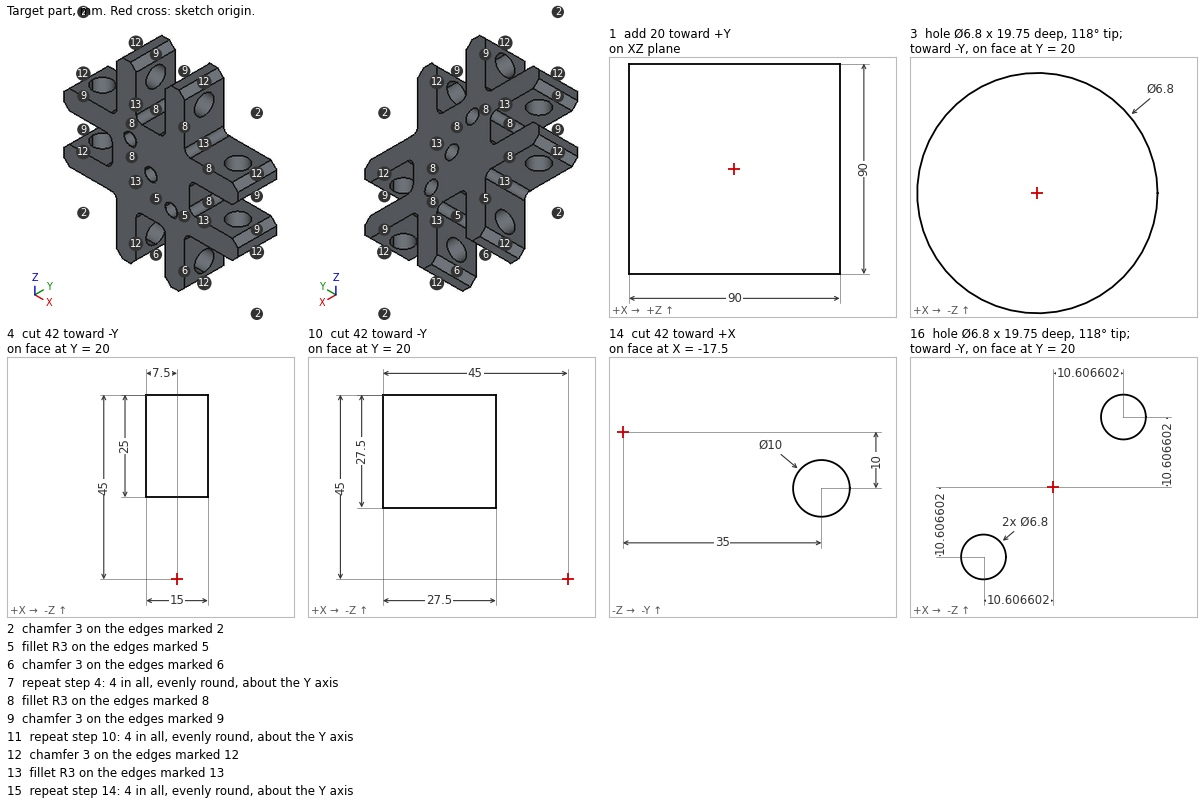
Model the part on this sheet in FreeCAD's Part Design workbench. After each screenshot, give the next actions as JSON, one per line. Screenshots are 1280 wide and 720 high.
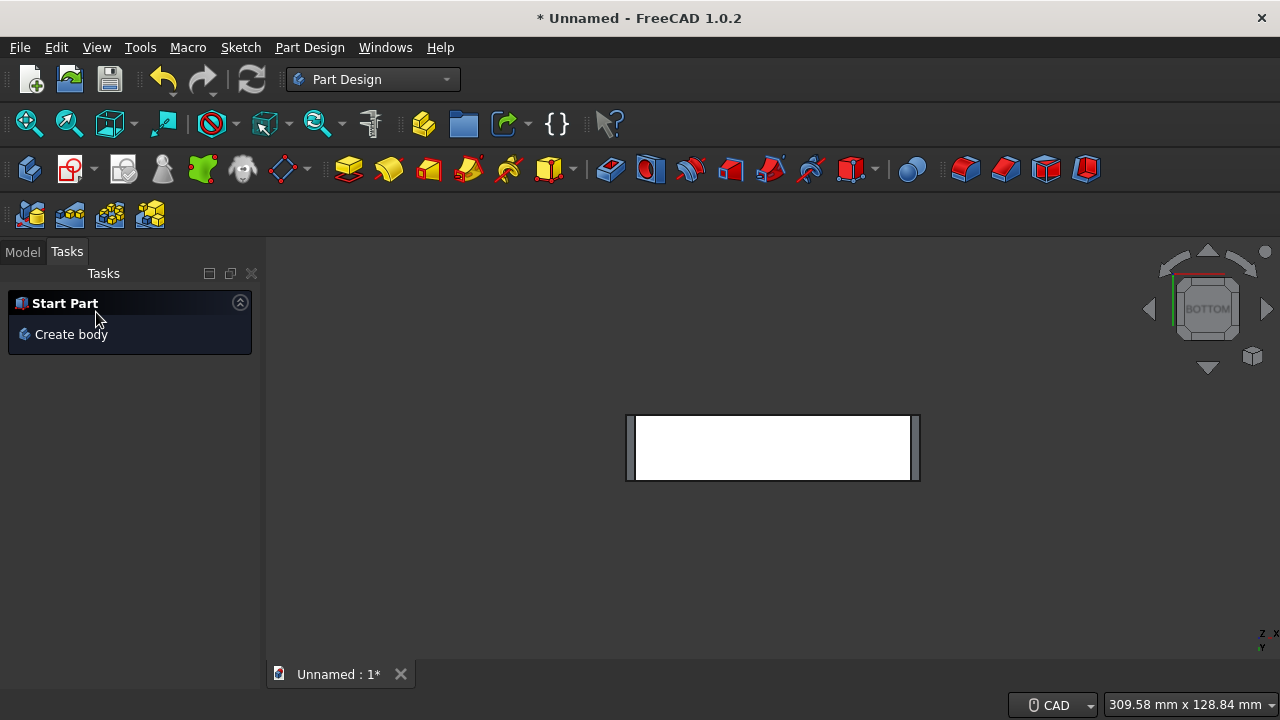
{"action": "left_click", "coordinate": [30, 124]}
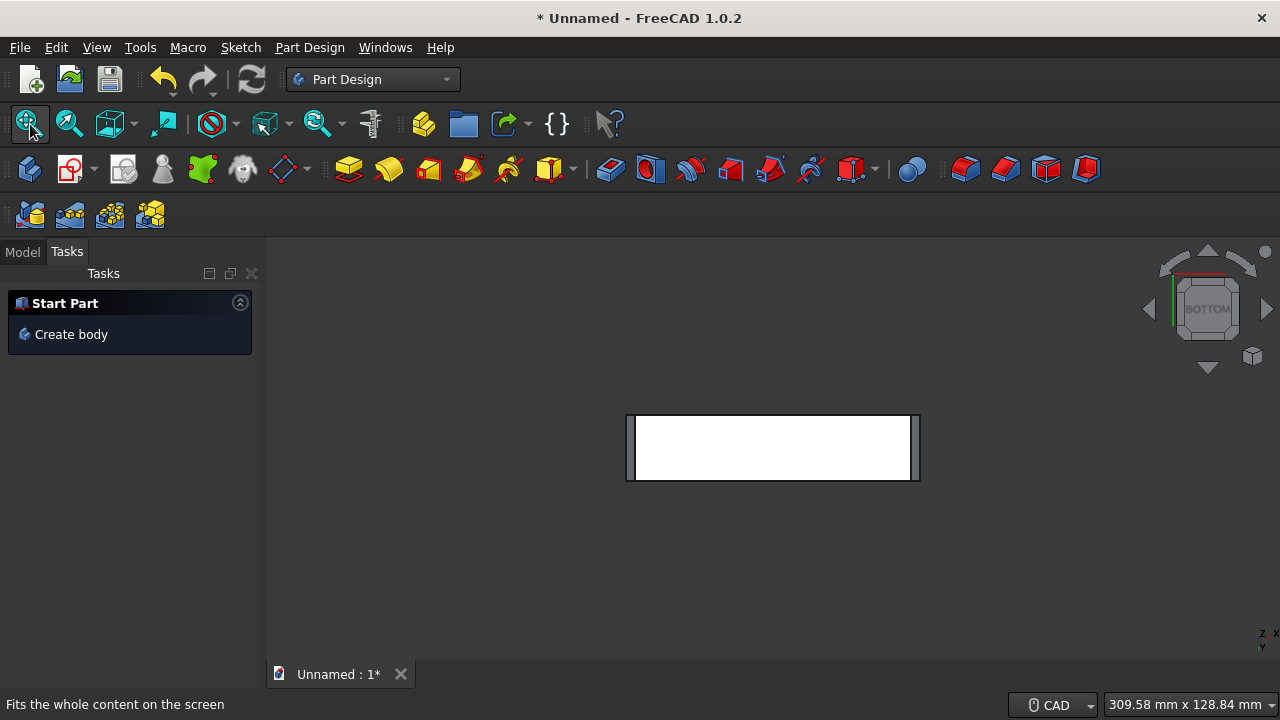
{"action": "key", "text": "4"}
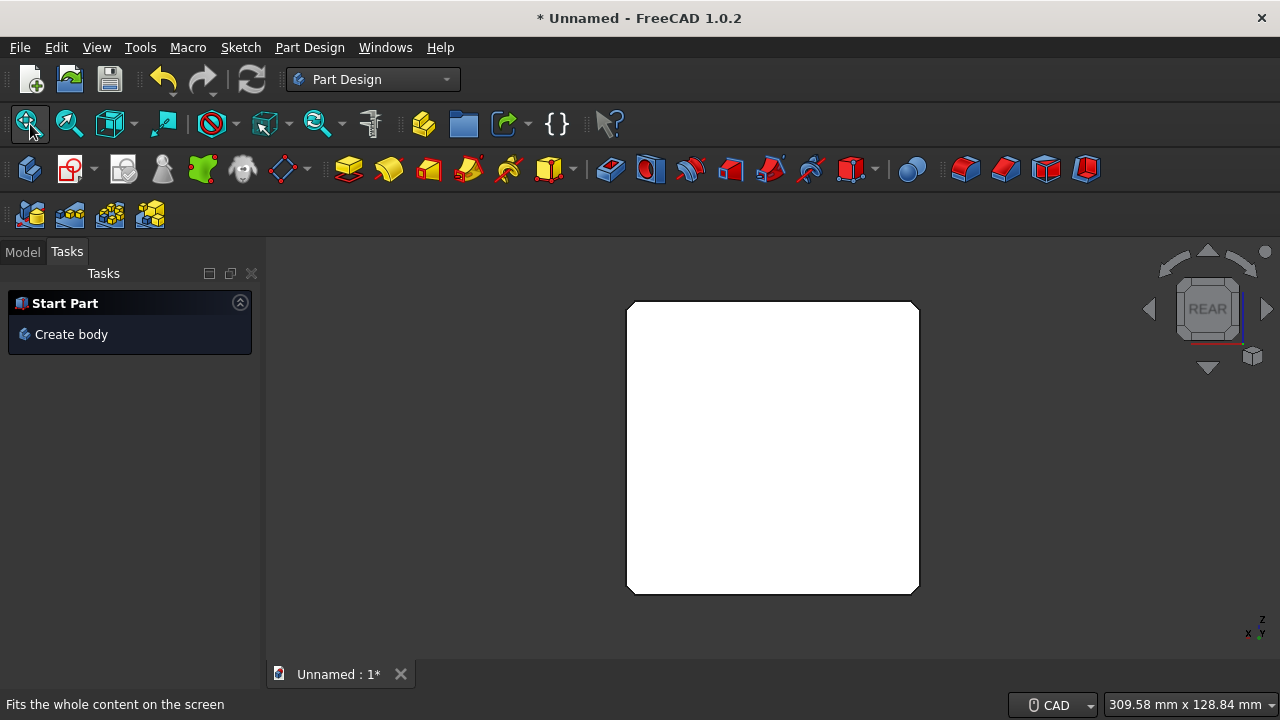
{"action": "left_click", "coordinate": [773, 447]}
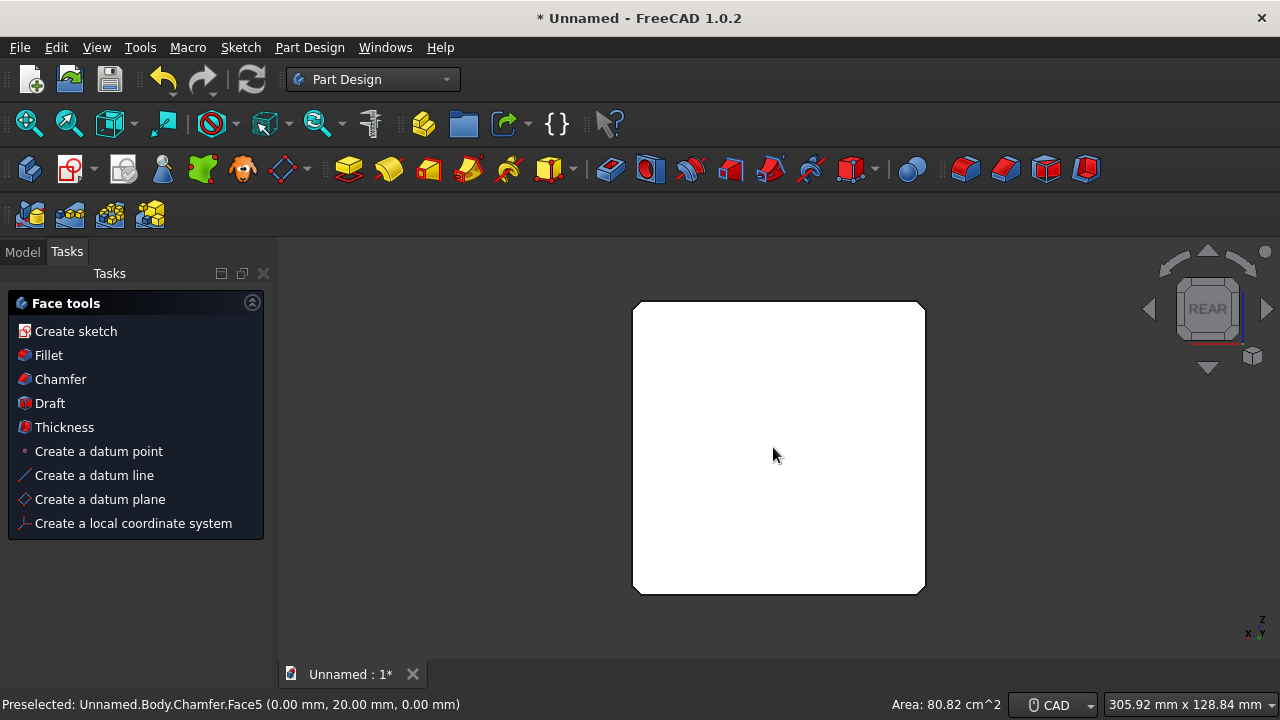
{"action": "left_click", "coordinate": [70, 170]}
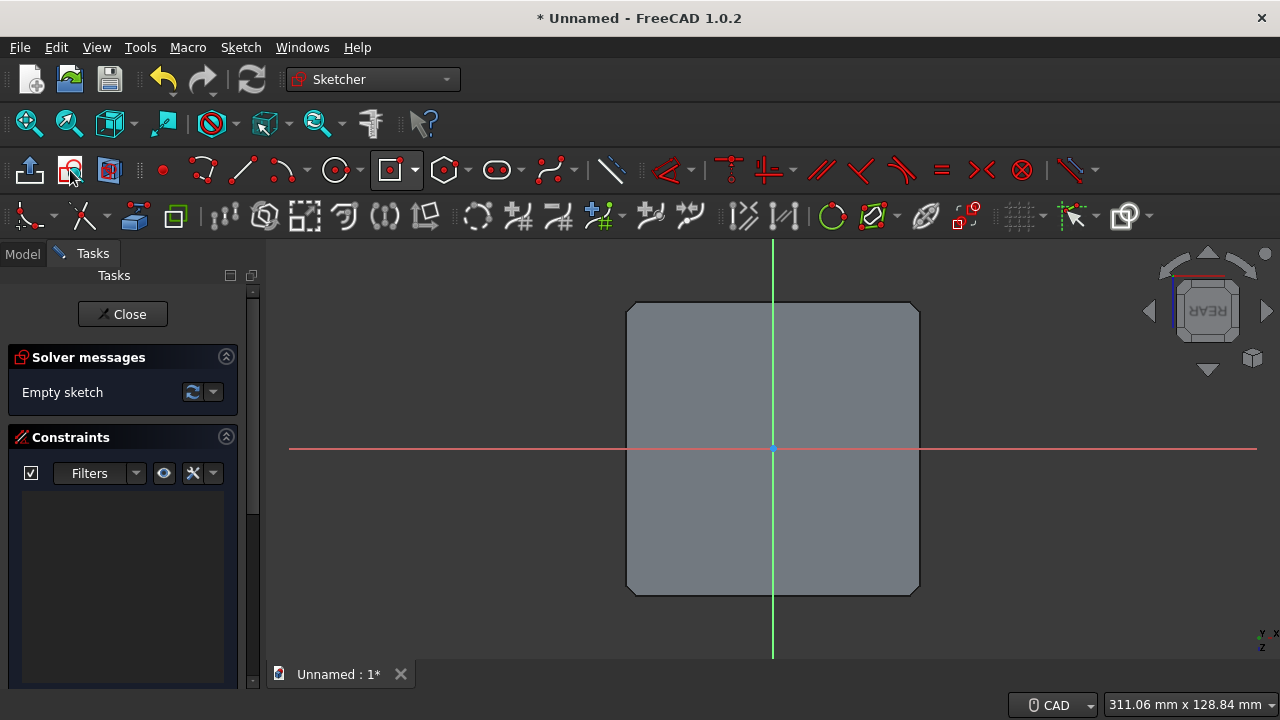
{"action": "scroll", "coordinate": [780, 449], "scroll_direction": "up", "scroll_amount": 12}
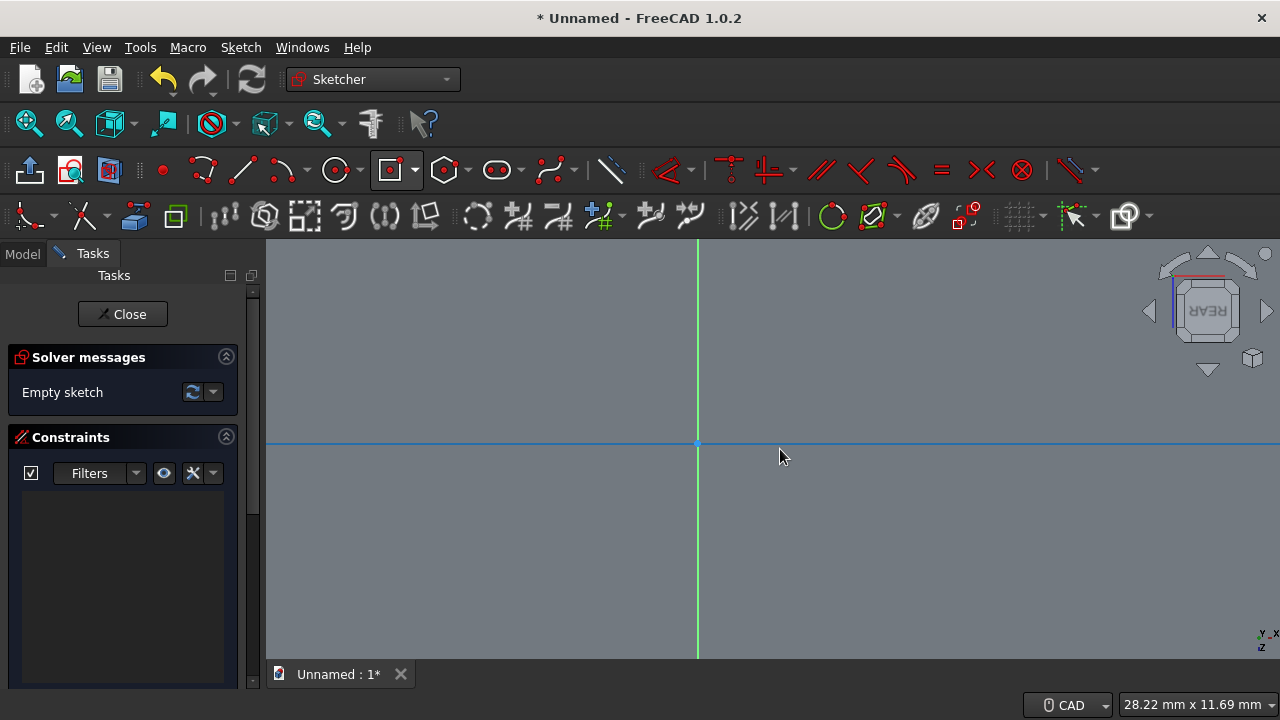
{"action": "left_click", "coordinate": [336, 170]}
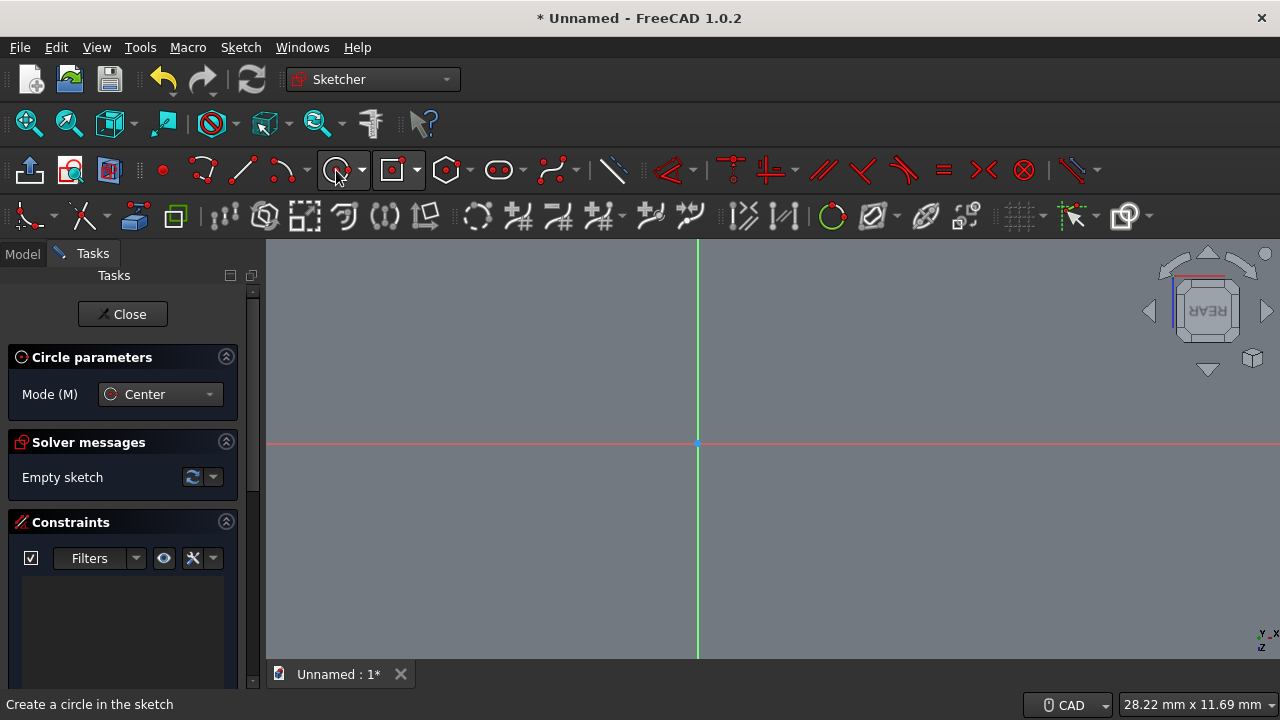
{"action": "left_click", "coordinate": [698, 444]}
{"action": "left_click", "coordinate": [784, 358]}
{"action": "key", "text": "Escape"}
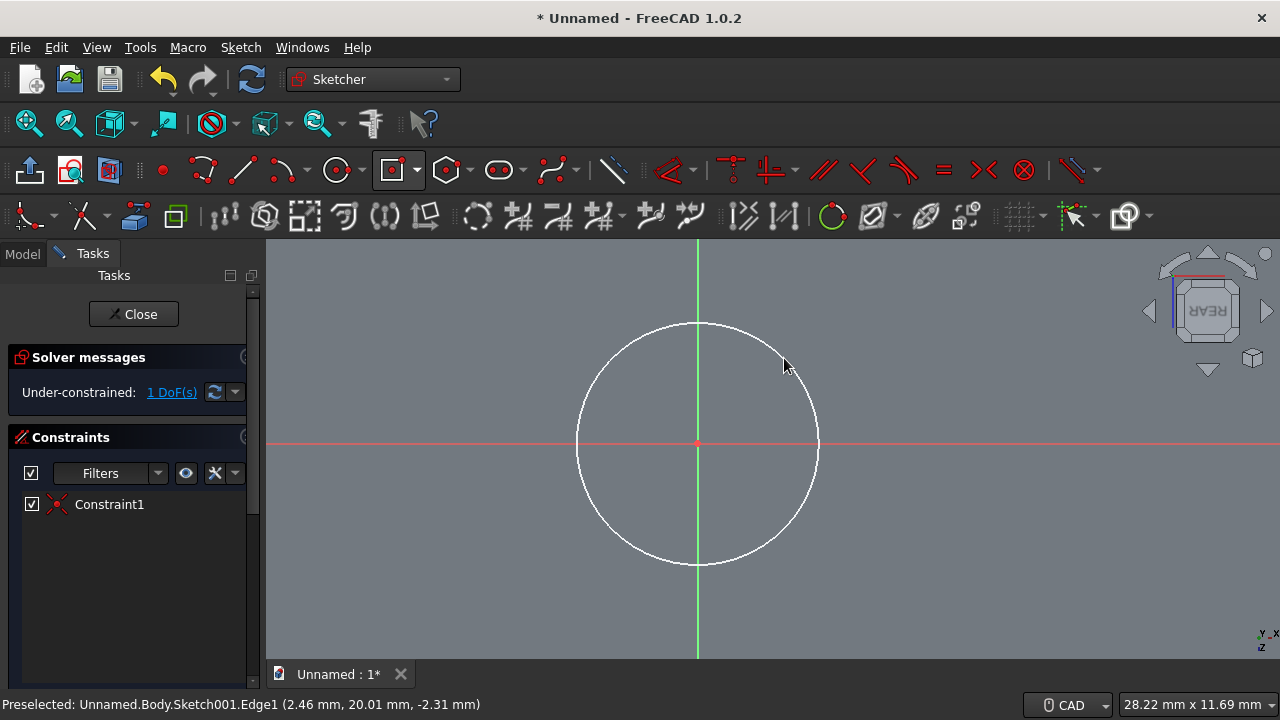
{"action": "left_click", "coordinate": [668, 170]}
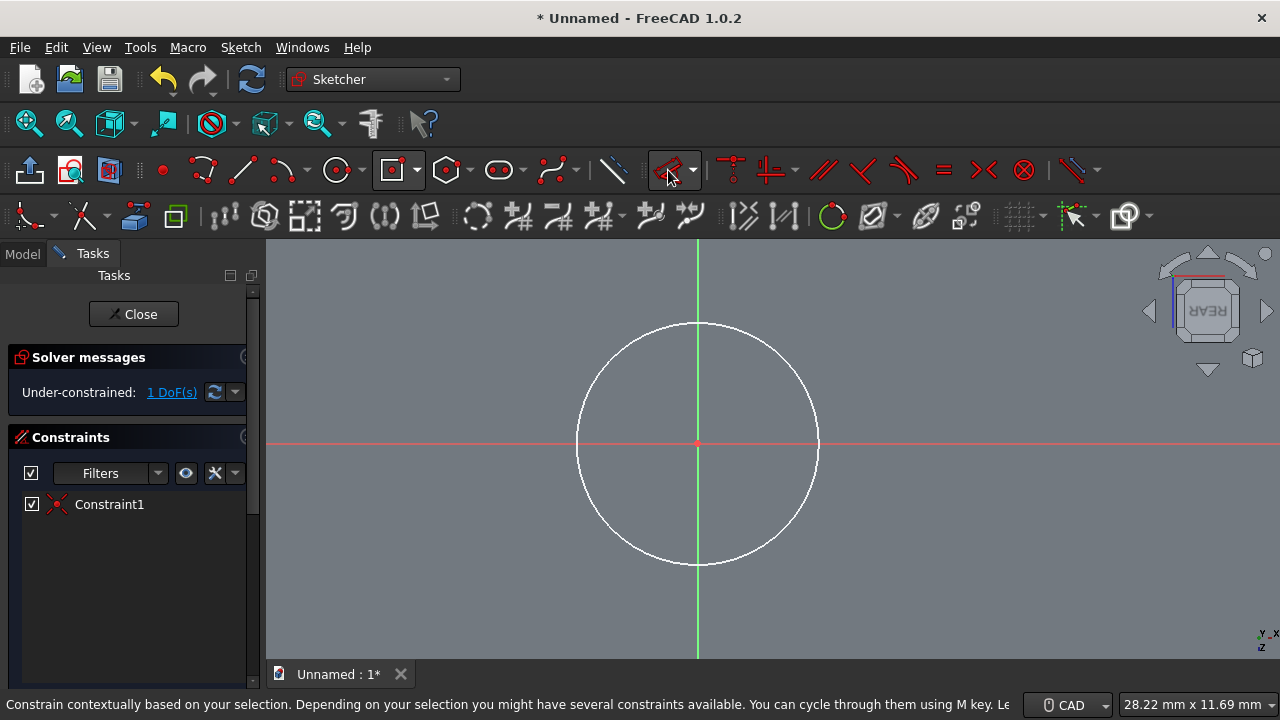
{"action": "left_click", "coordinate": [783, 358]}
{"action": "left_click", "coordinate": [806, 335]}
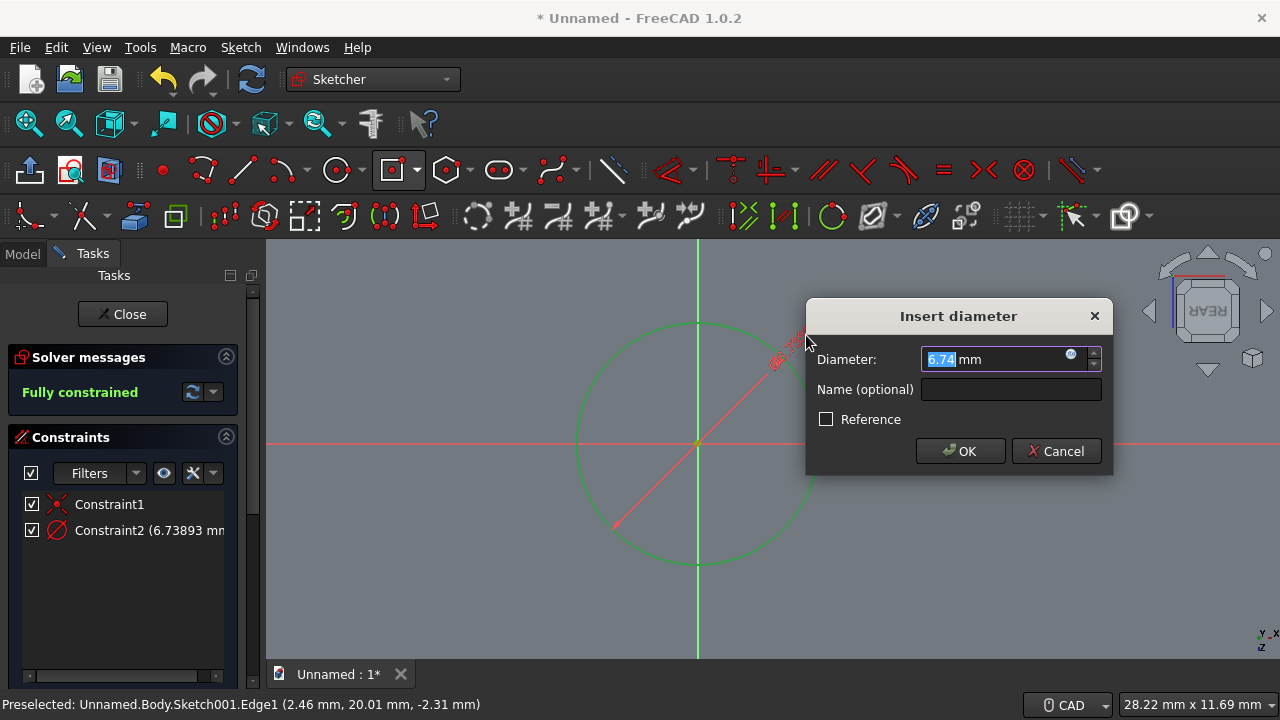
{"action": "type", "text": "6.8"}
{"action": "key", "text": "Return"}
{"action": "key", "text": "Escape"}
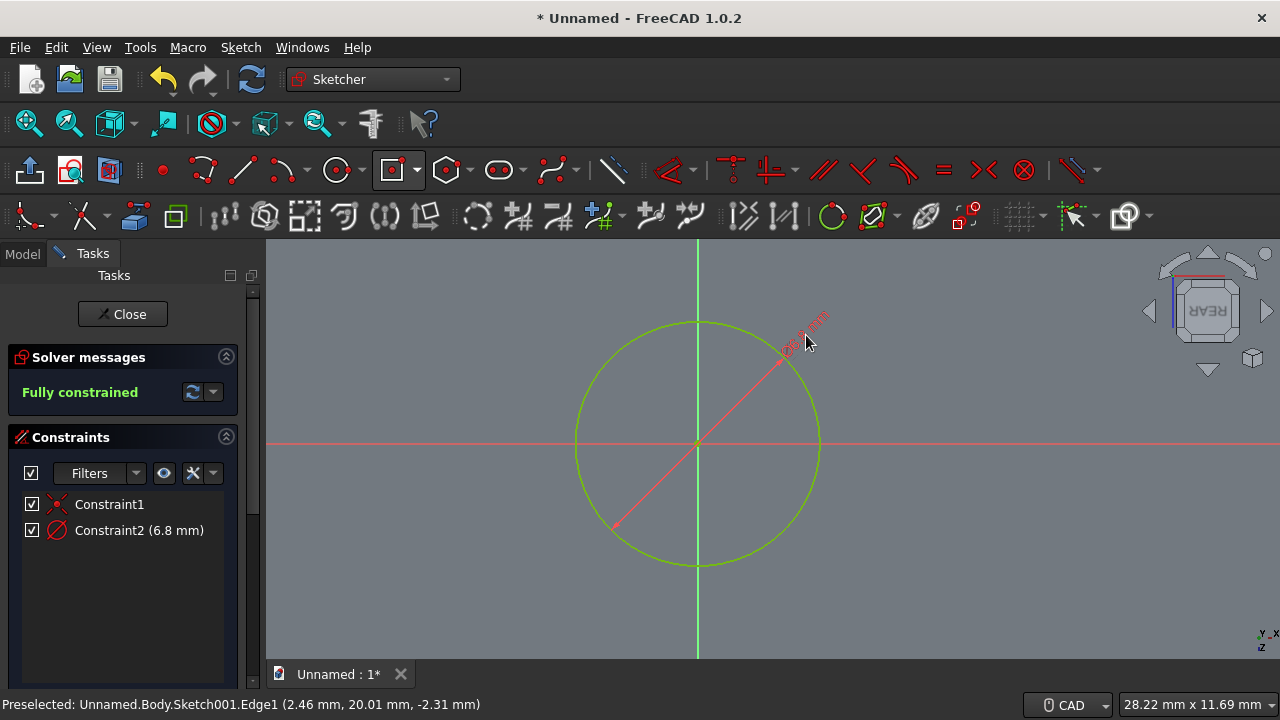
{"action": "left_click", "coordinate": [123, 314]}